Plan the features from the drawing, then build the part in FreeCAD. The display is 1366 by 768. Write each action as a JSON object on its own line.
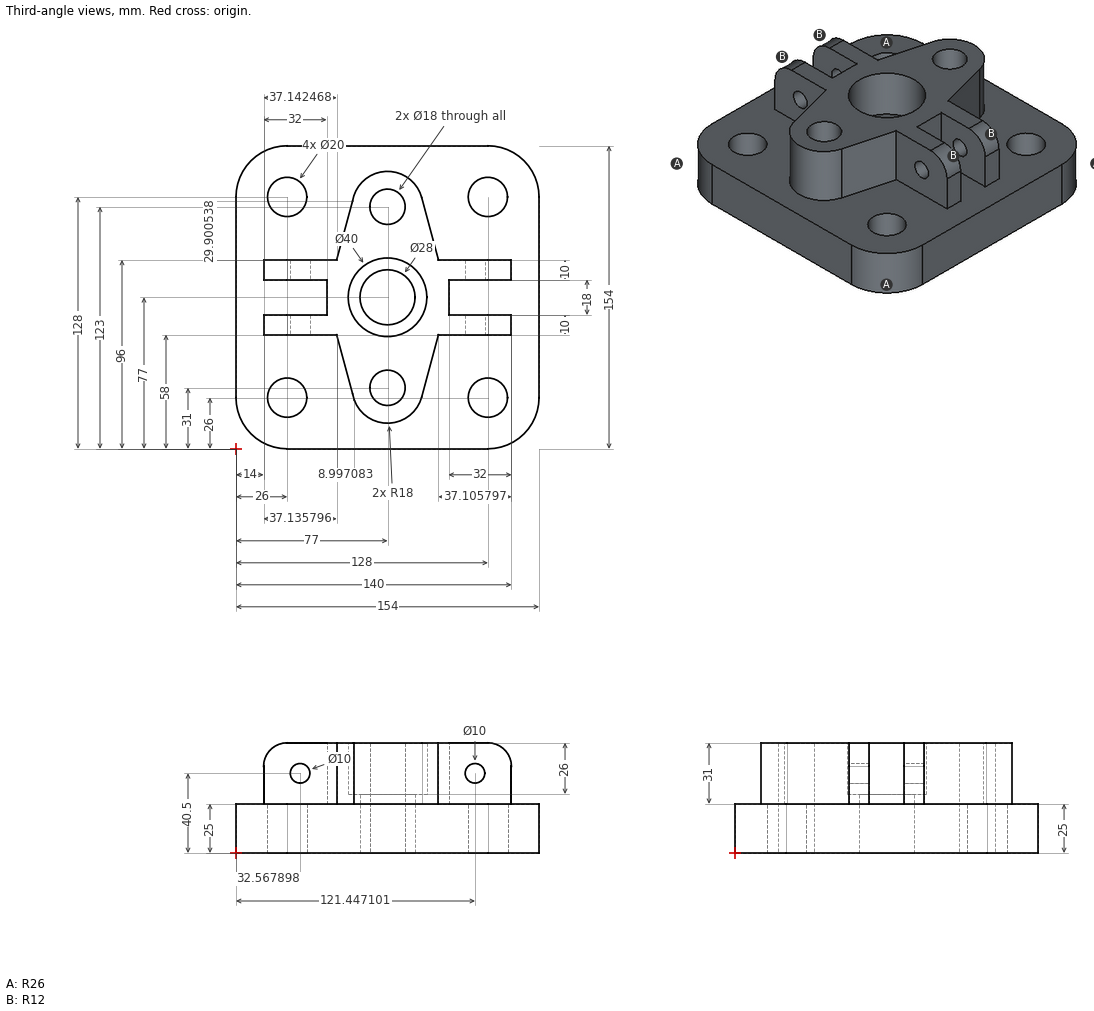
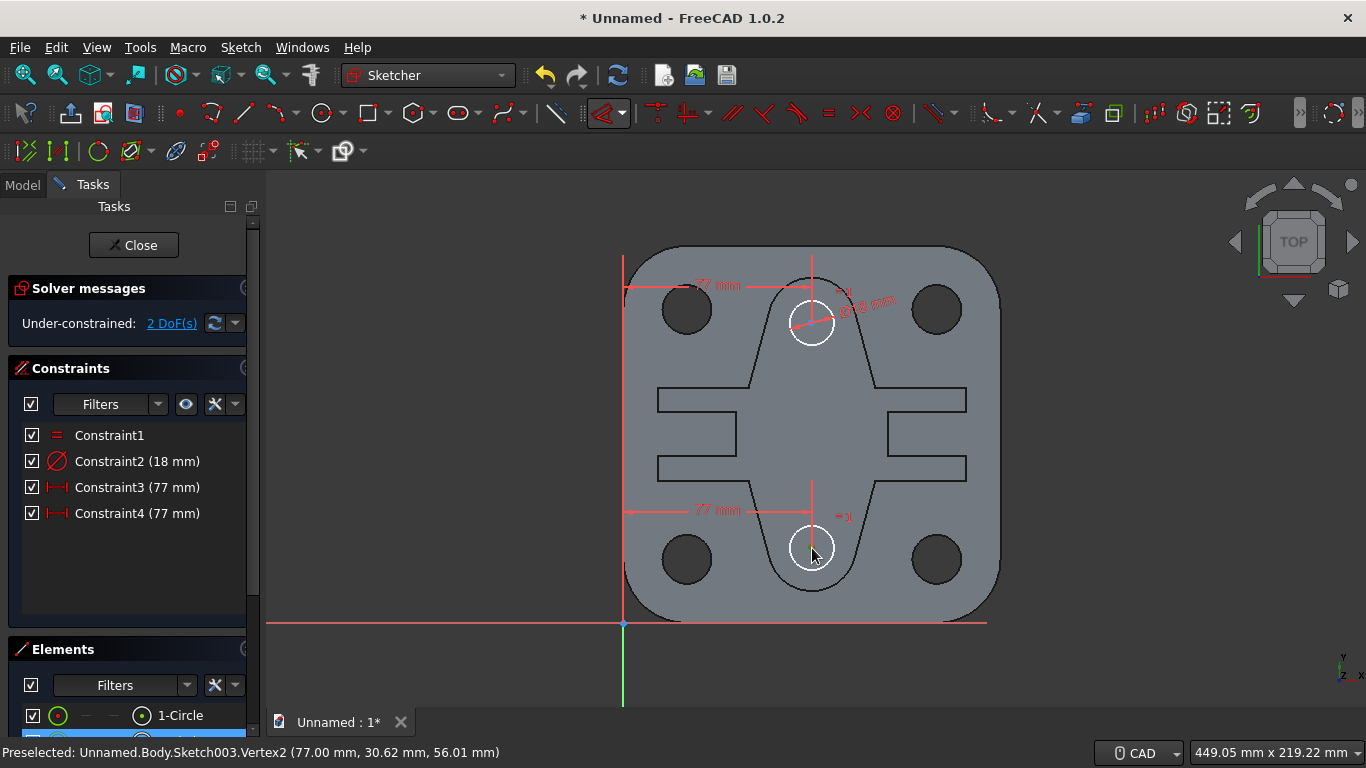
{"action": "left_click", "coordinate": [624, 114]}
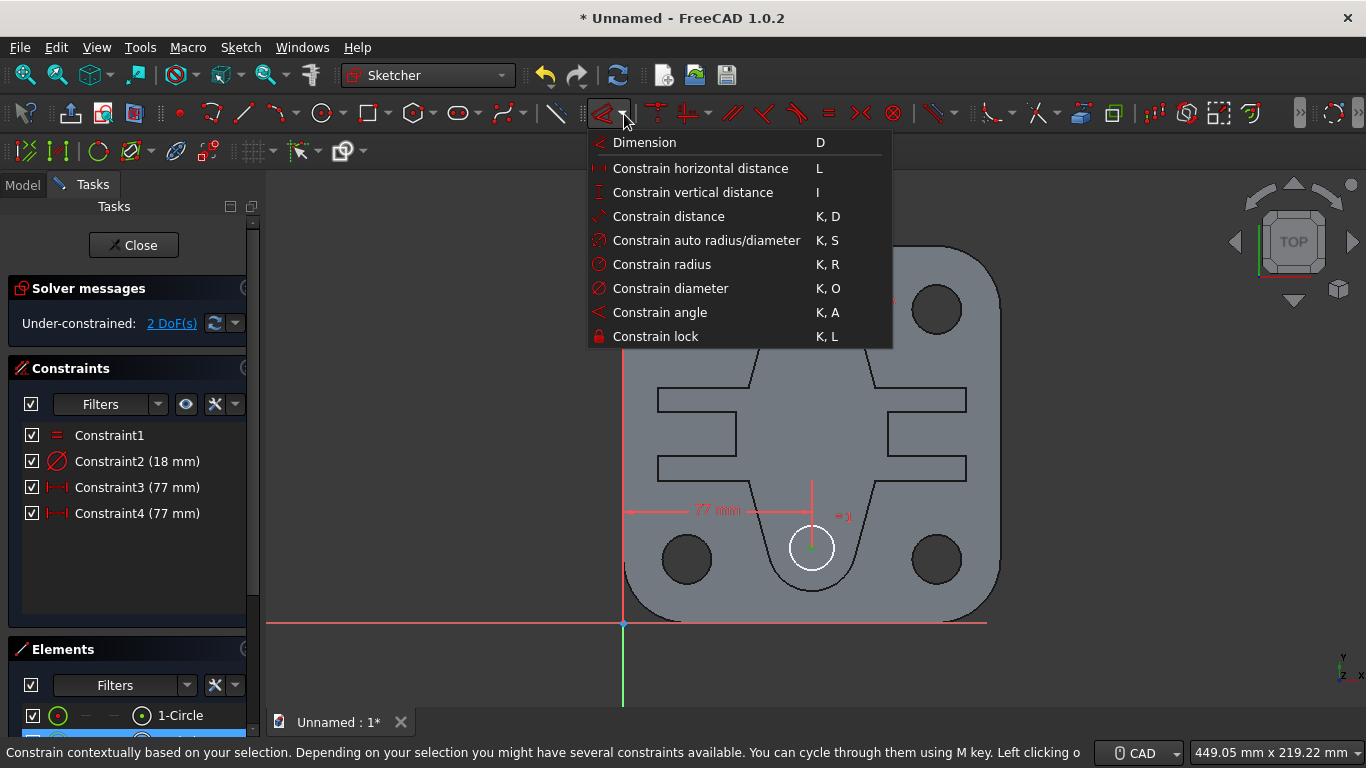
{"action": "left_click", "coordinate": [740, 192]}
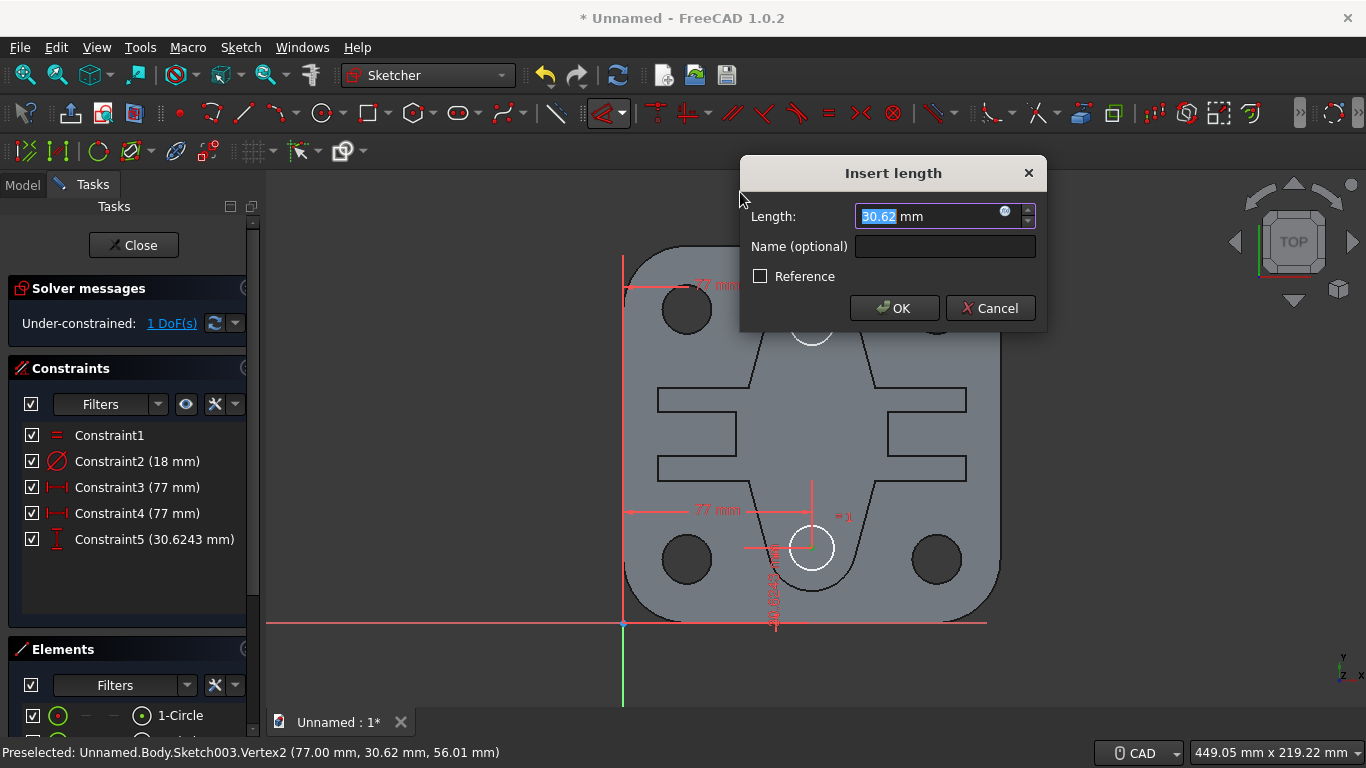
{"action": "type", "text": "31"}
{"action": "key", "text": "Return"}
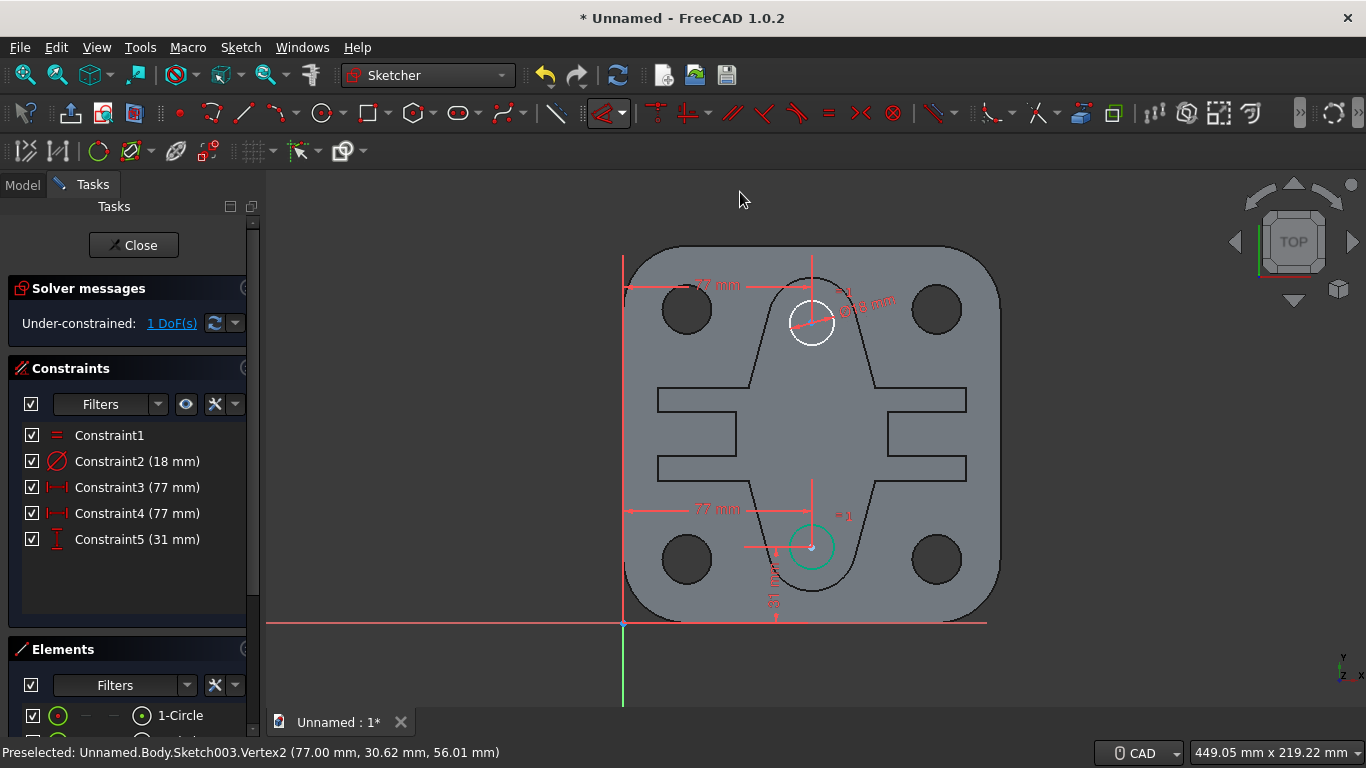
{"action": "left_click", "coordinate": [812, 323]}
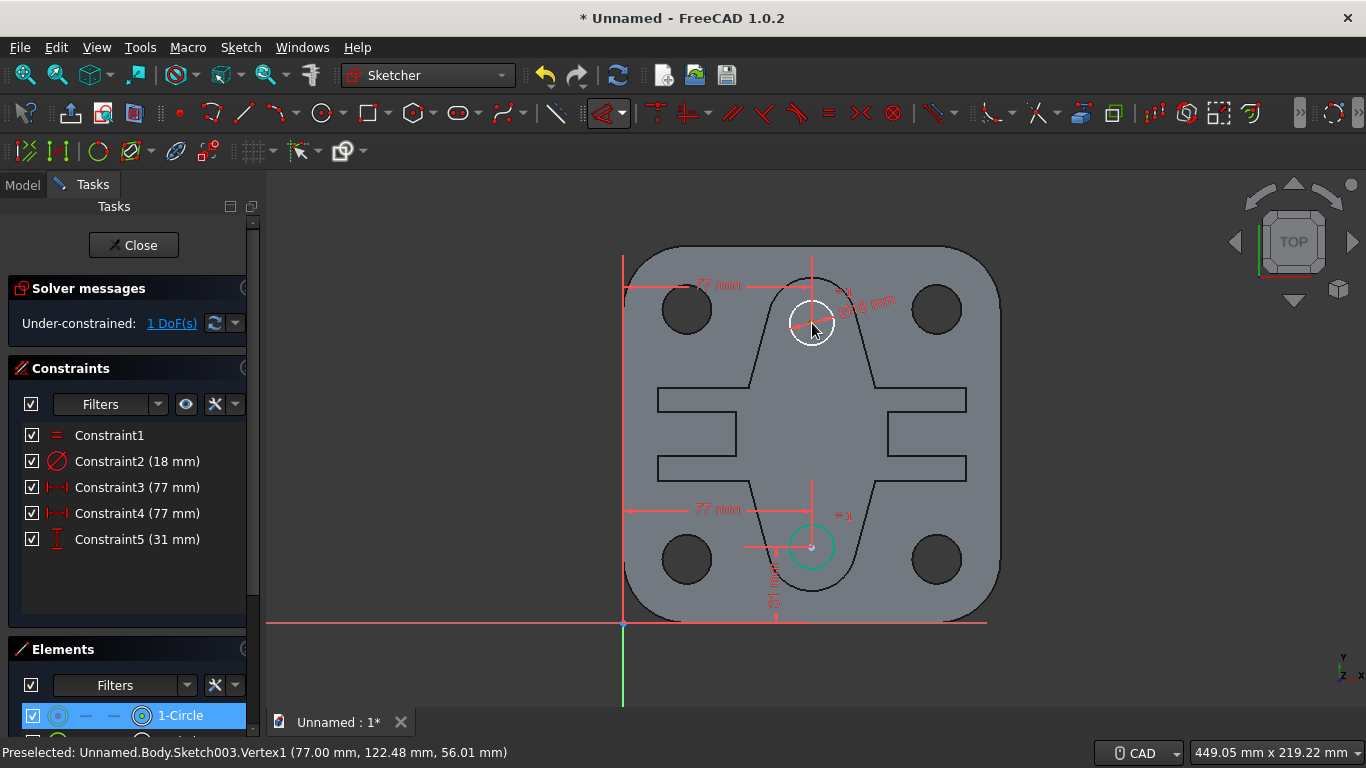
{"action": "left_click", "coordinate": [624, 114]}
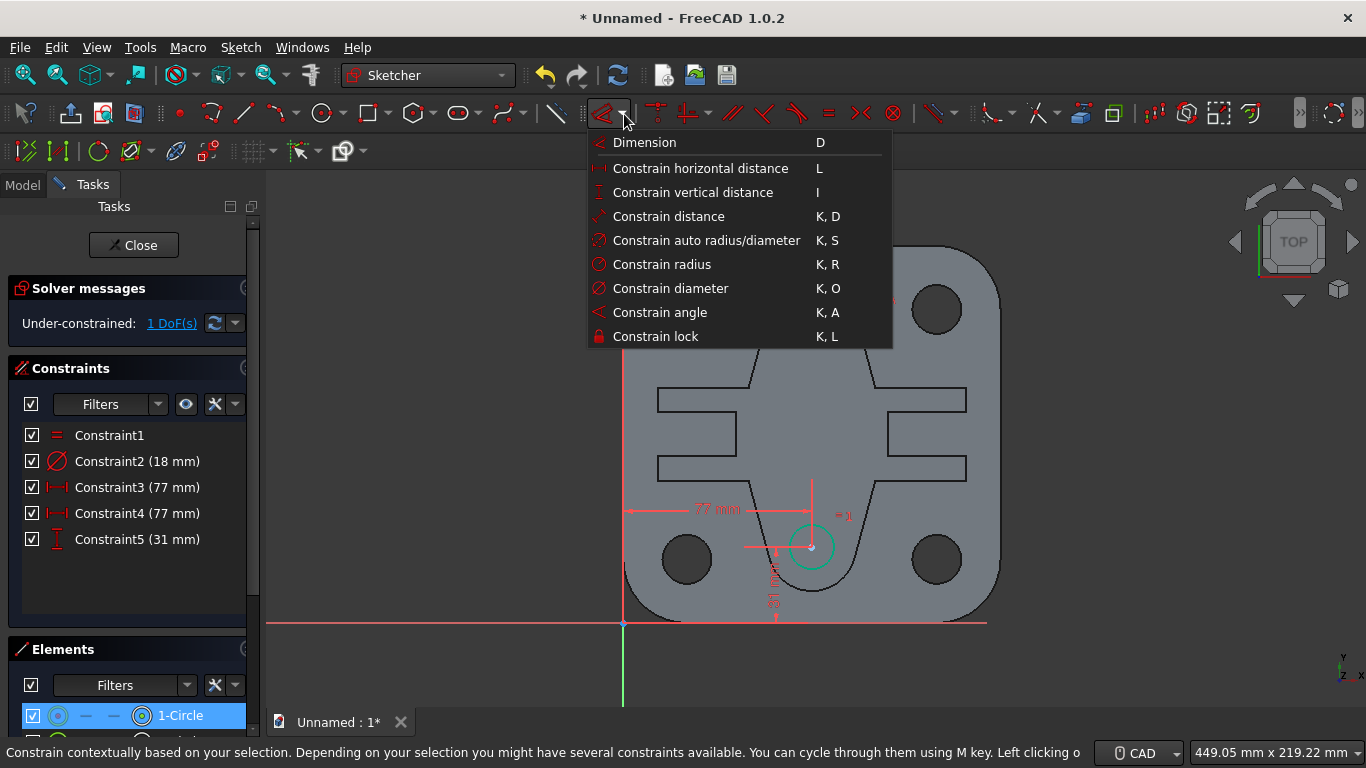
{"action": "left_click", "coordinate": [740, 192]}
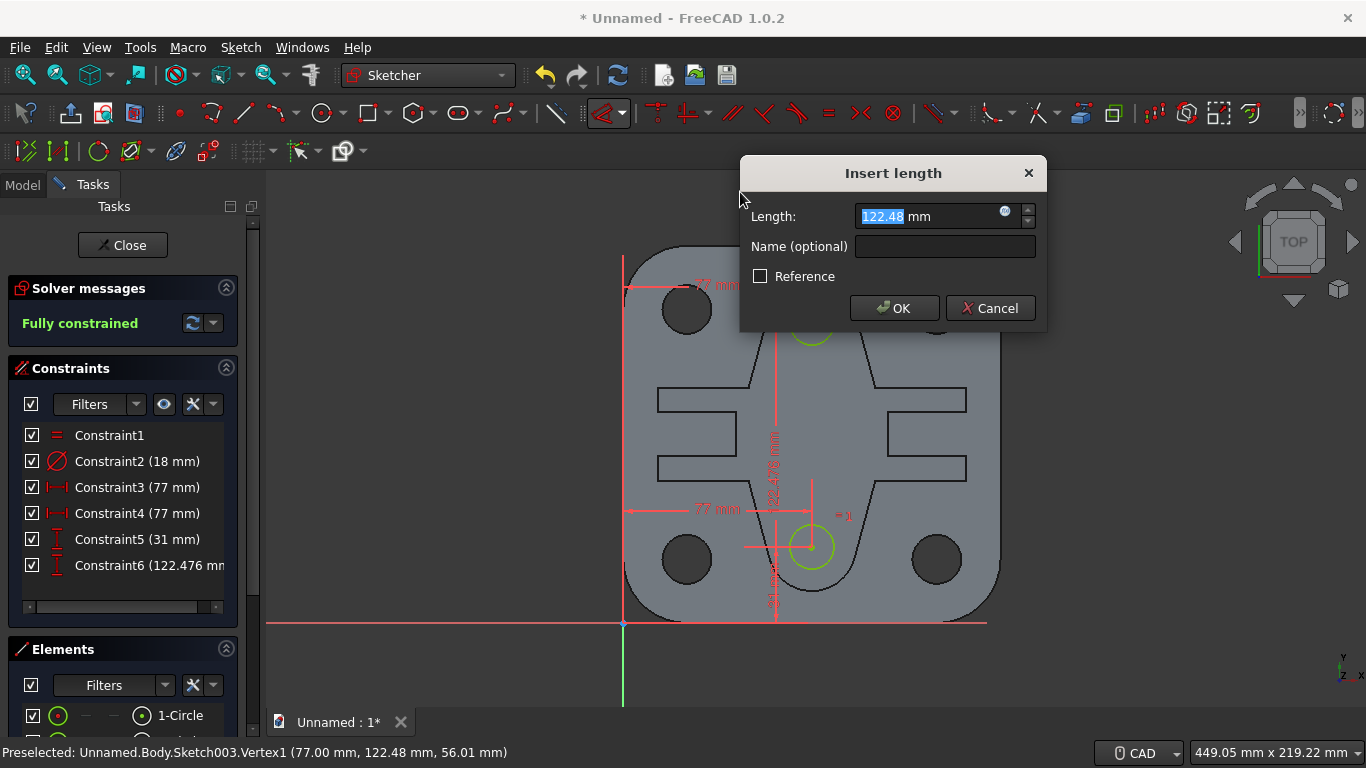
{"action": "type", "text": "123"}
{"action": "key", "text": "Return"}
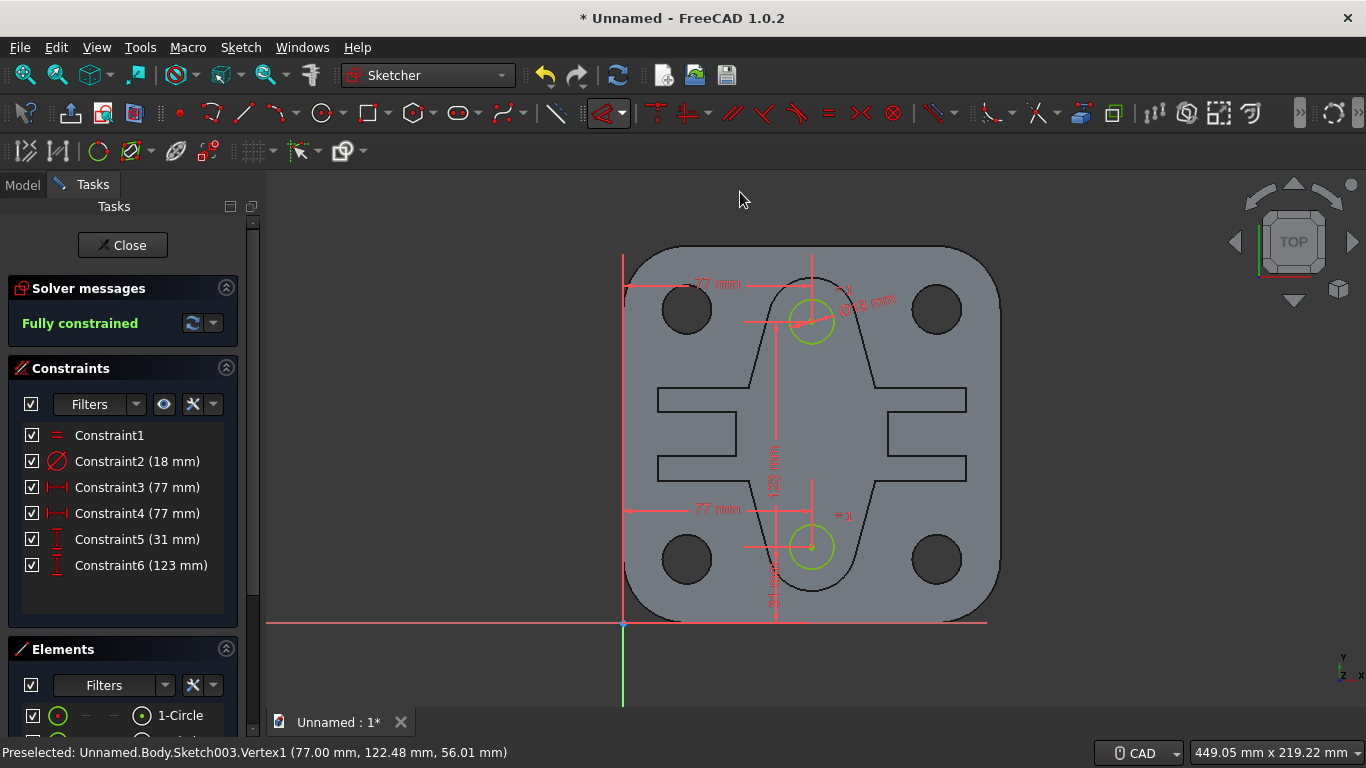
{"action": "left_click", "coordinate": [123, 245]}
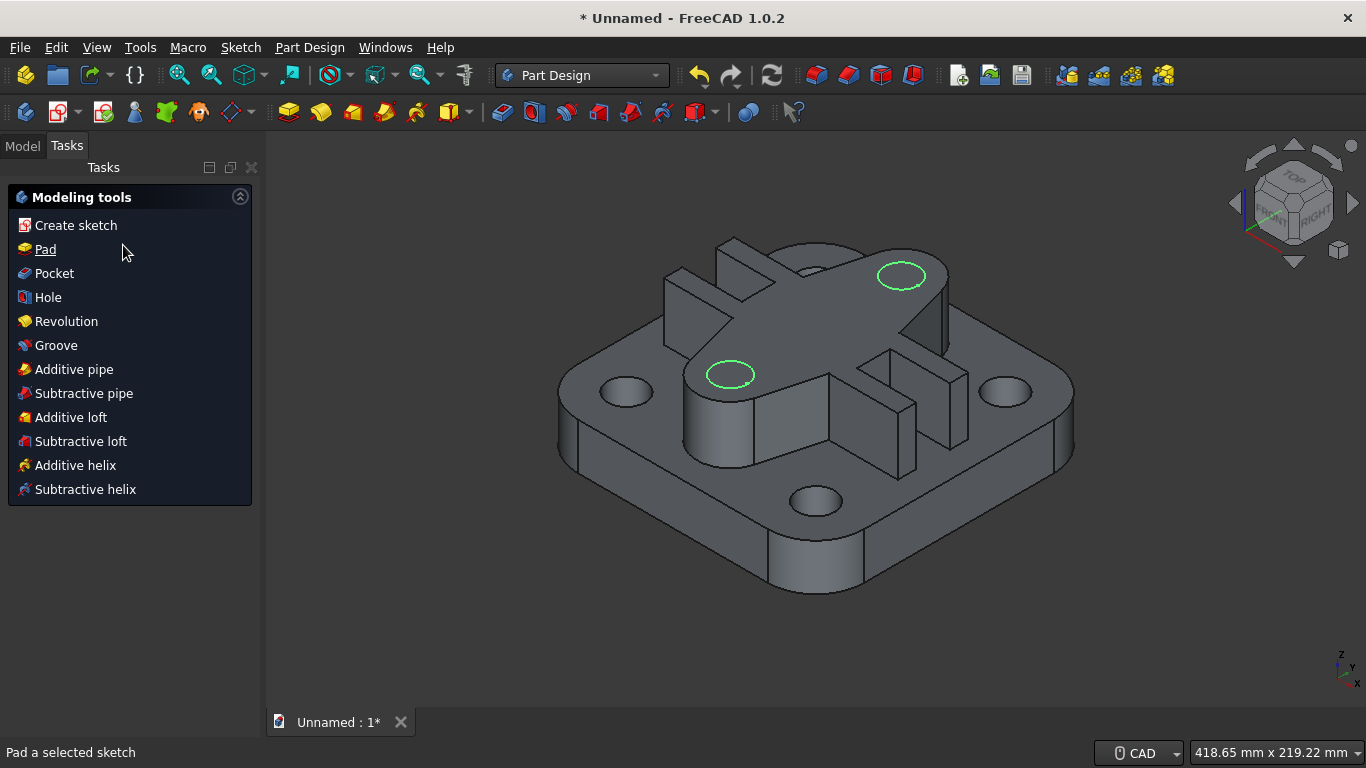
{"action": "left_click", "coordinate": [536, 112]}